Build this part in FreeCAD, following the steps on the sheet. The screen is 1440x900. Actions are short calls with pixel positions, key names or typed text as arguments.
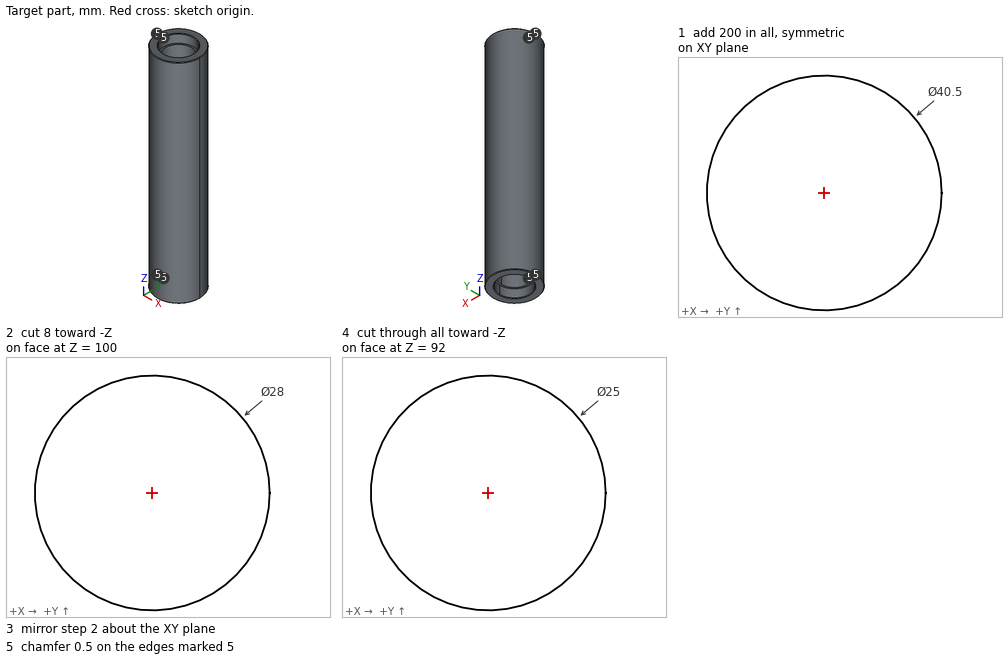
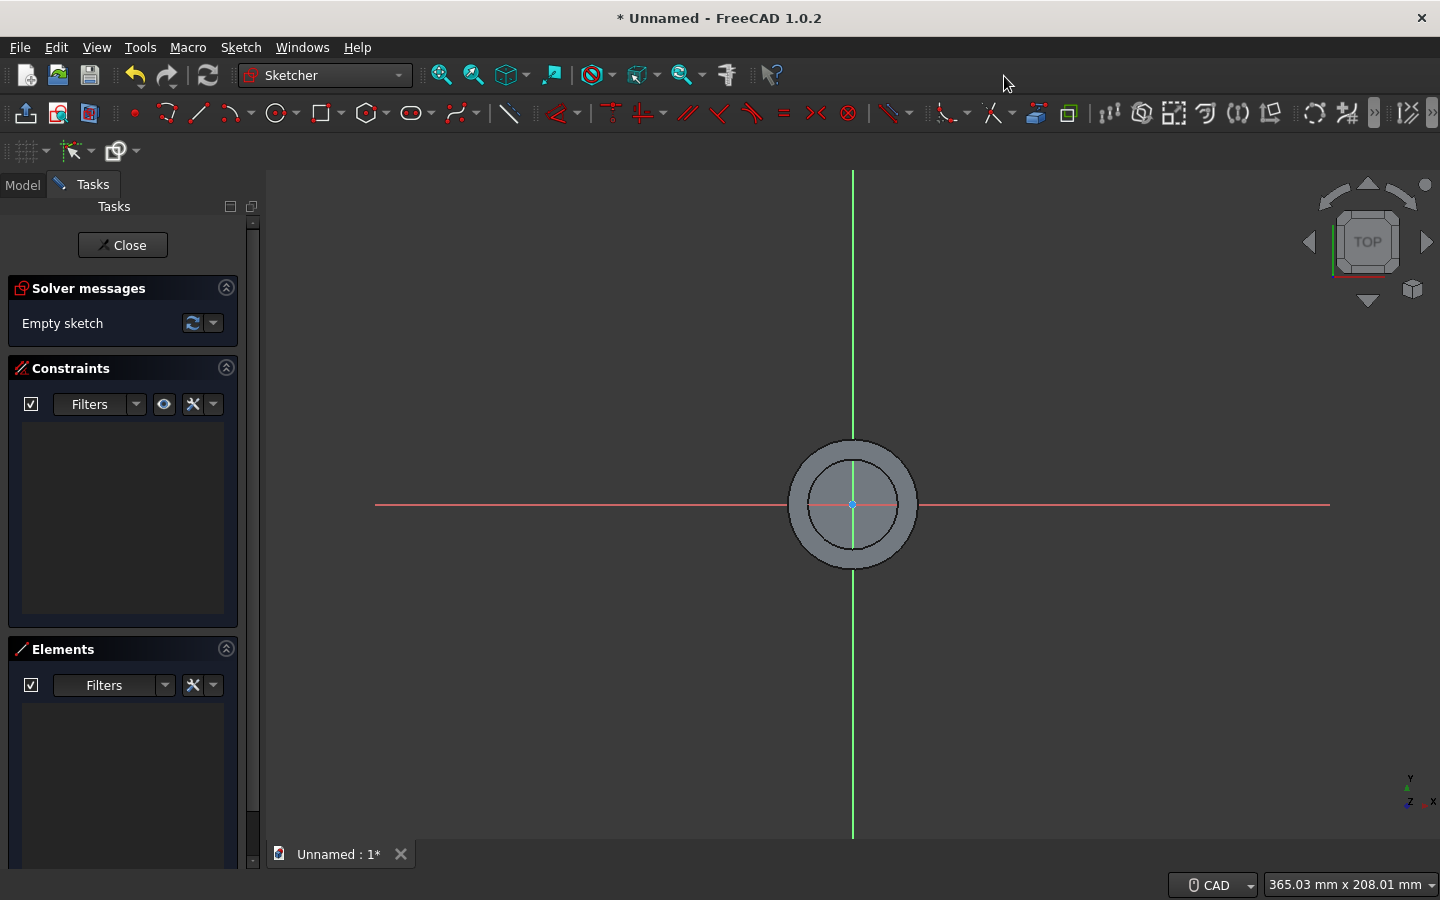
scroll(870, 504, up, 8)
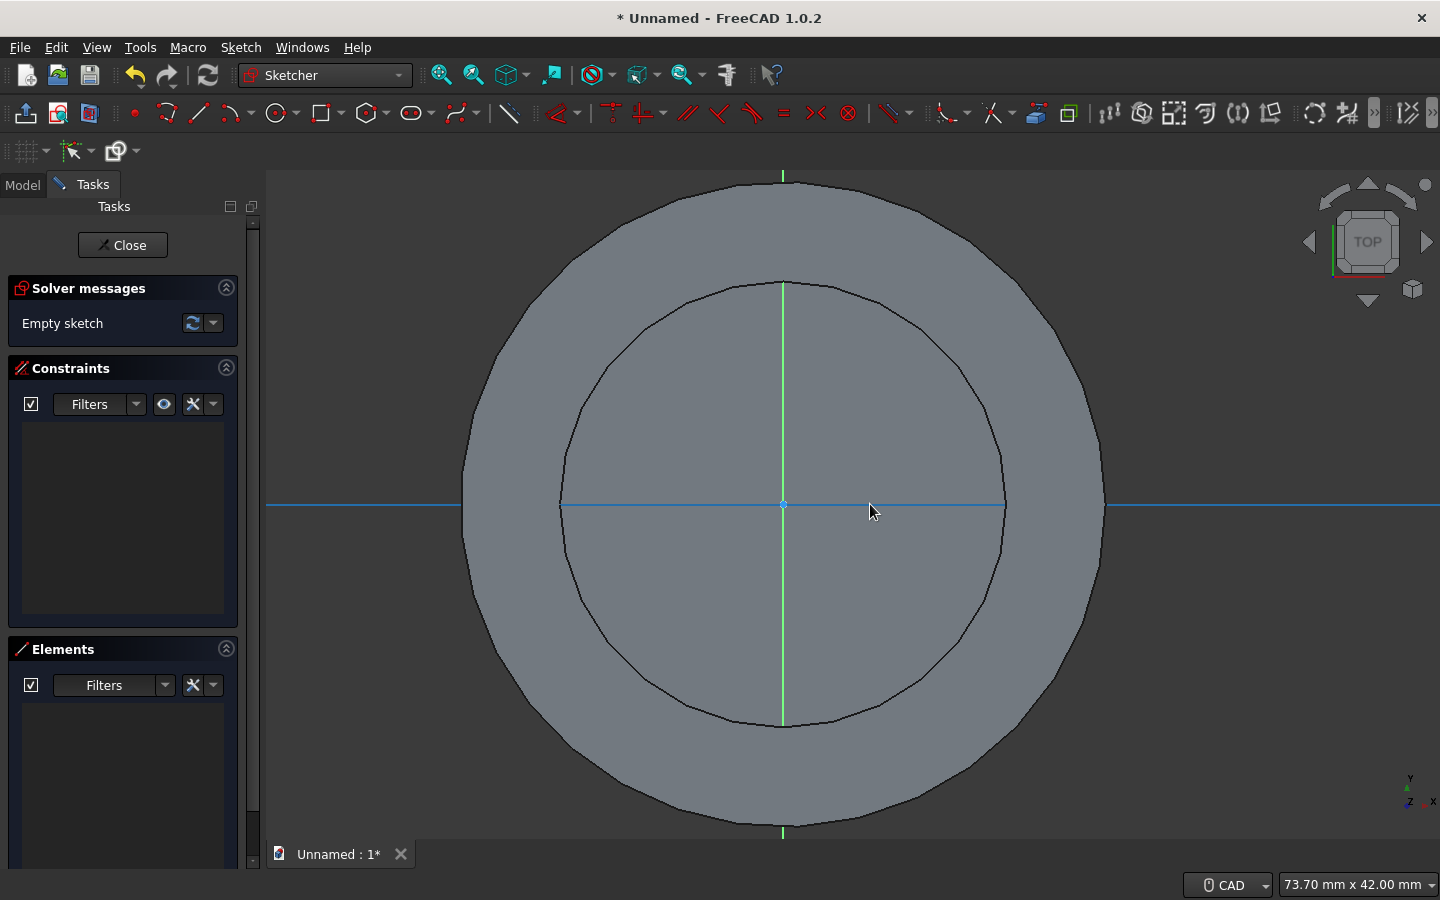
click(276, 114)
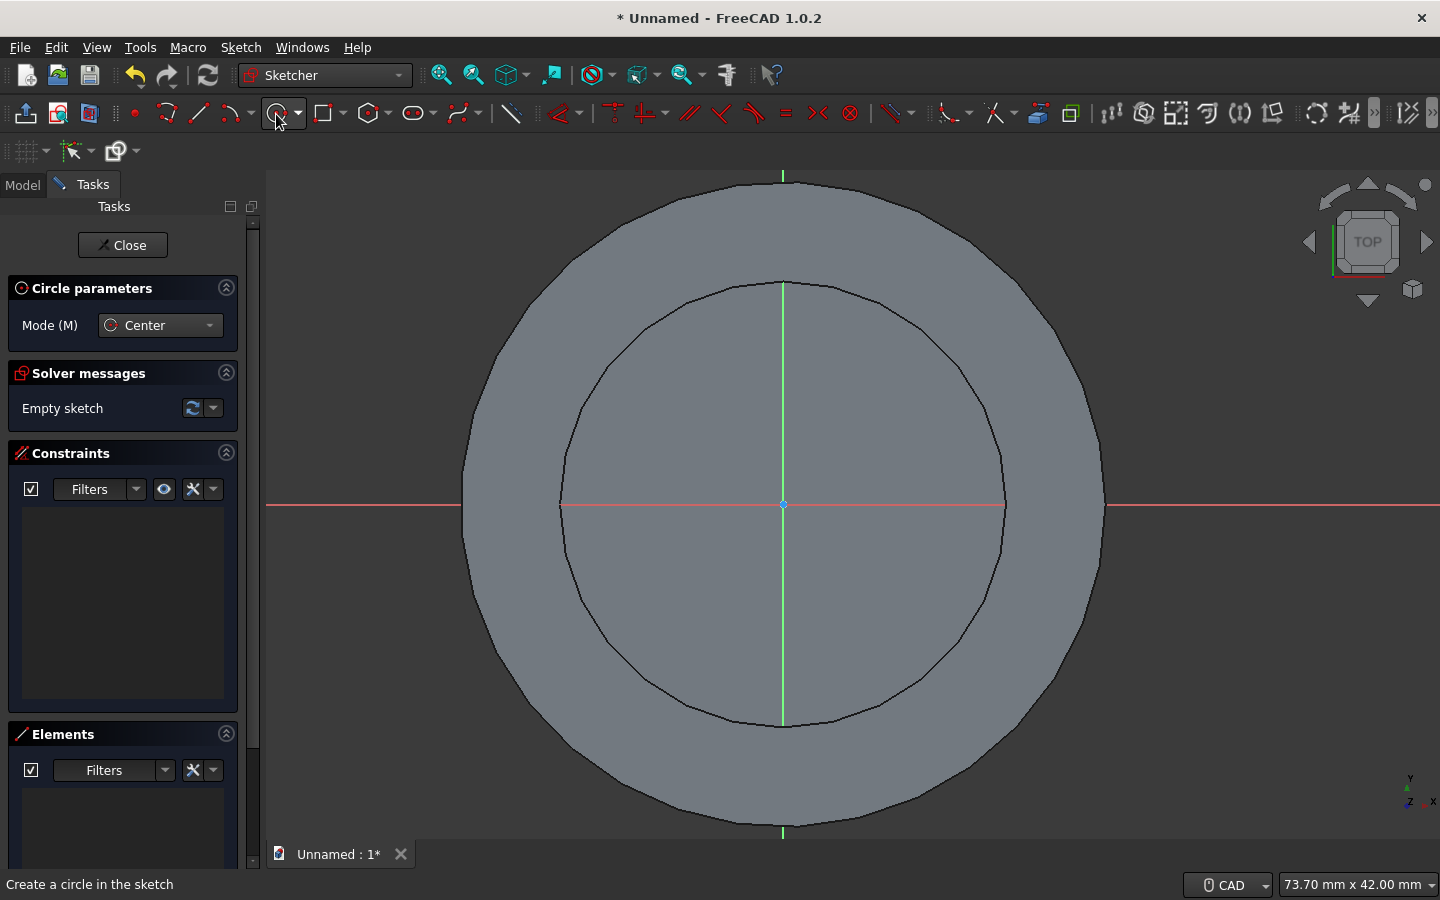
click(783, 504)
move(924, 364)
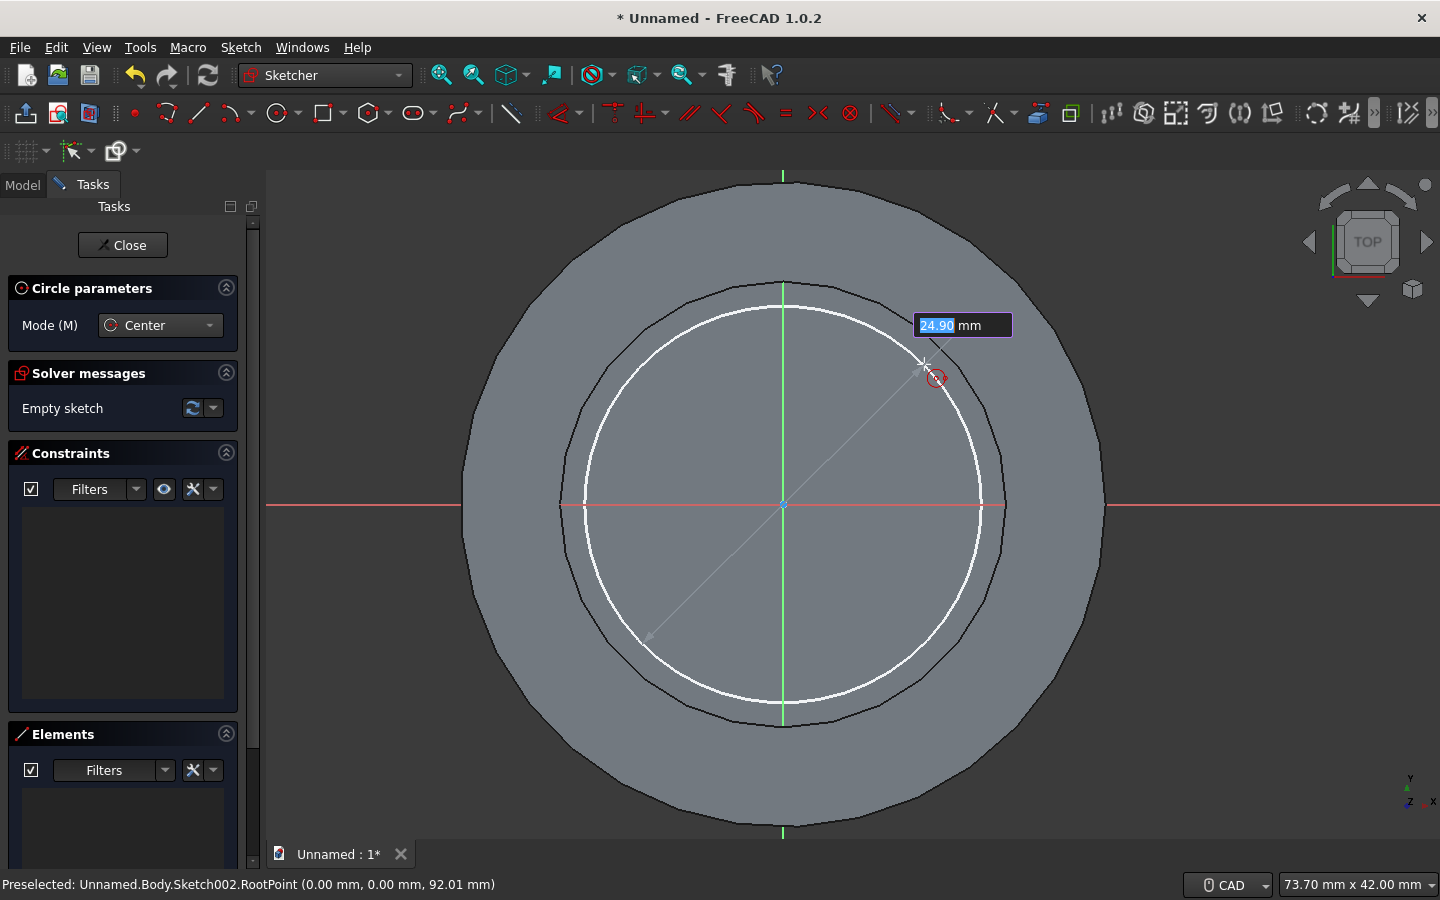
text(25)
key(Return)
key(Escape)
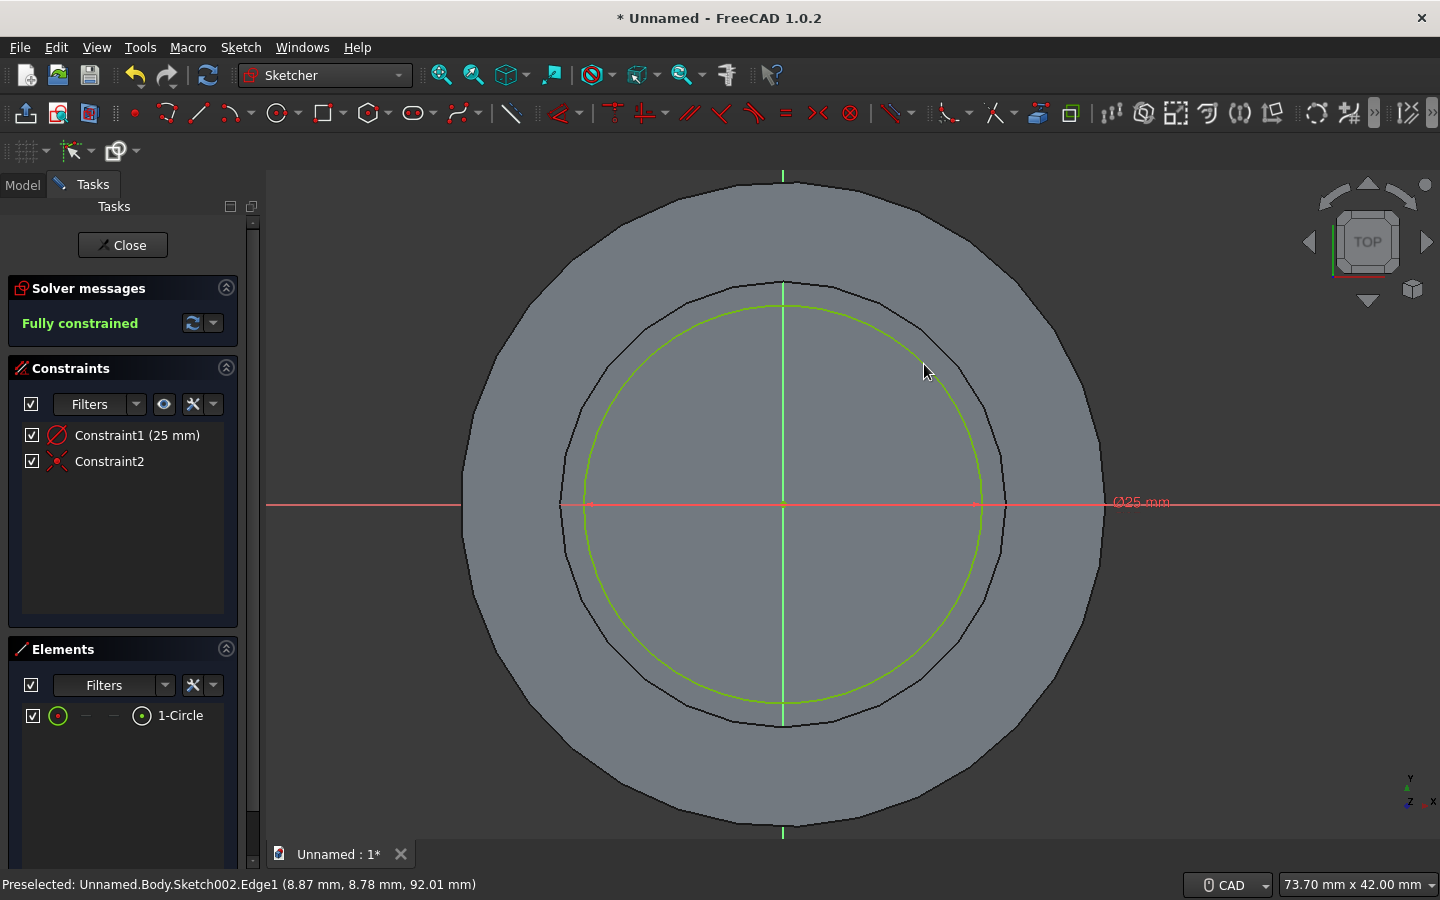
click(123, 245)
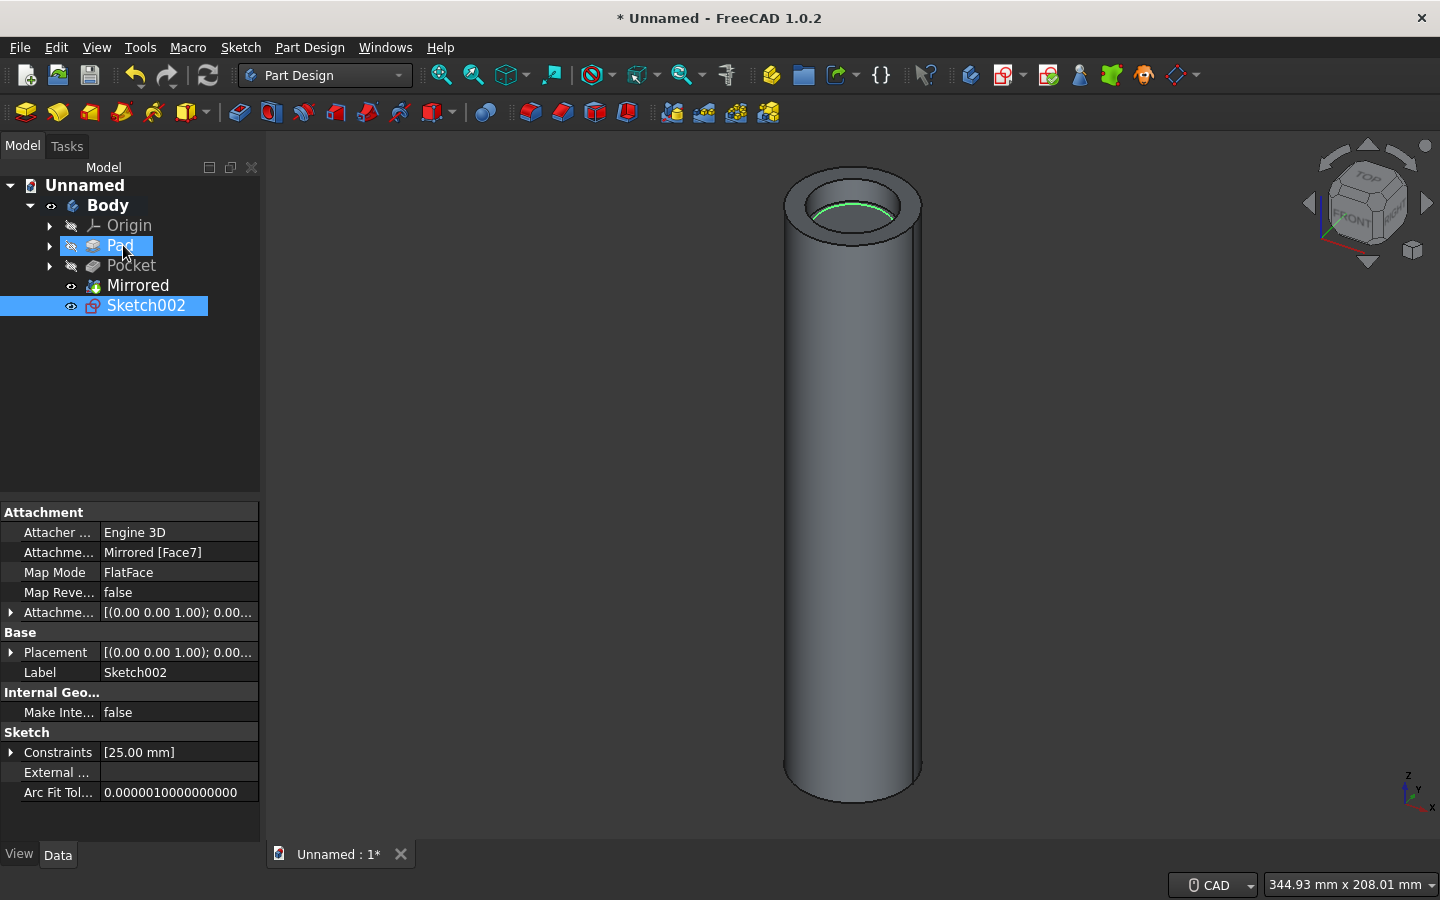
click(240, 112)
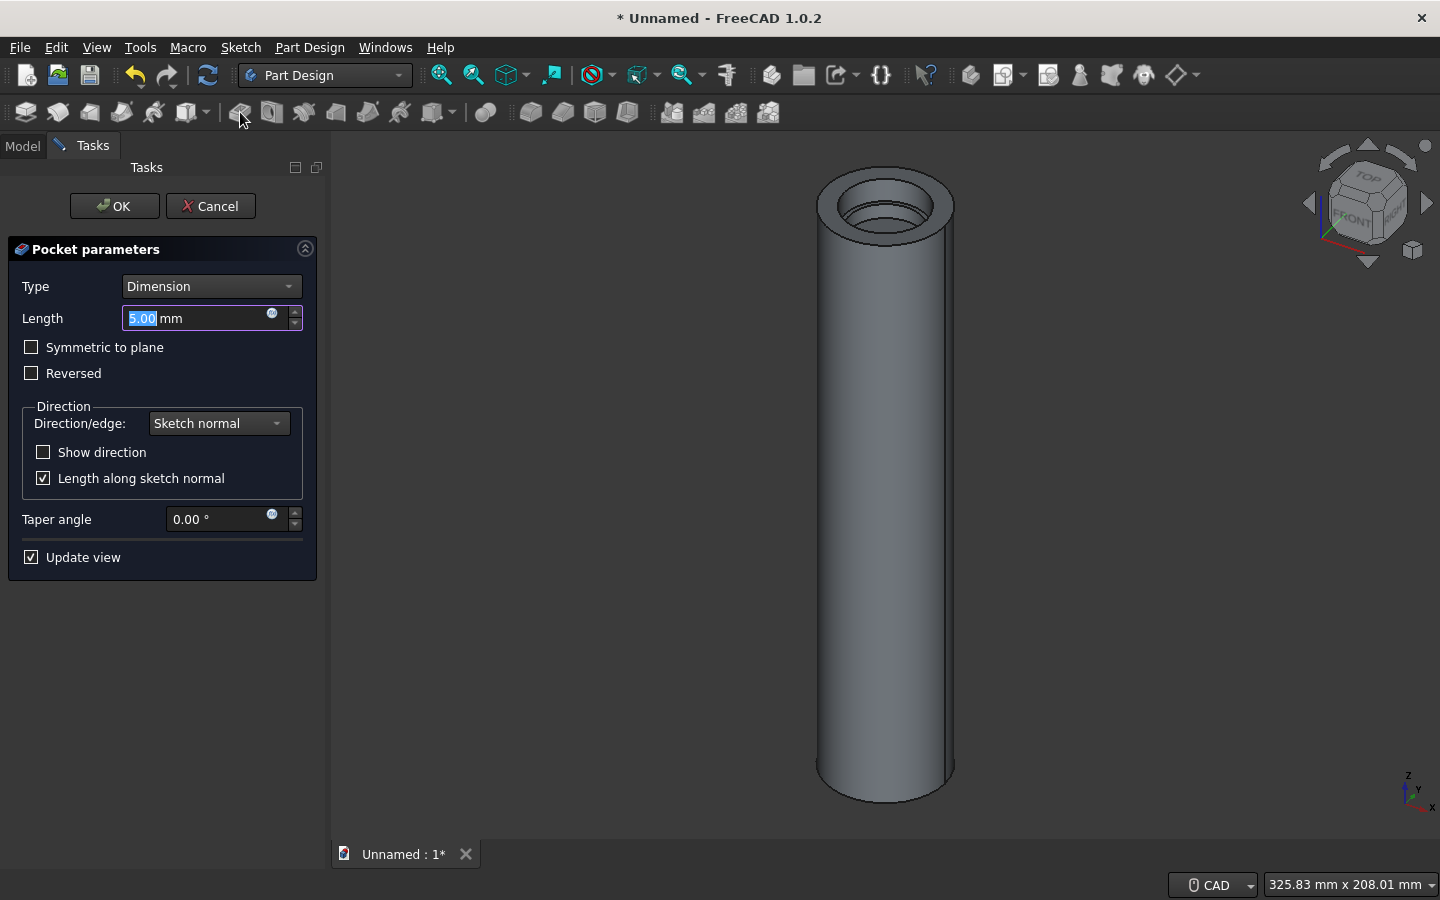
click(212, 286)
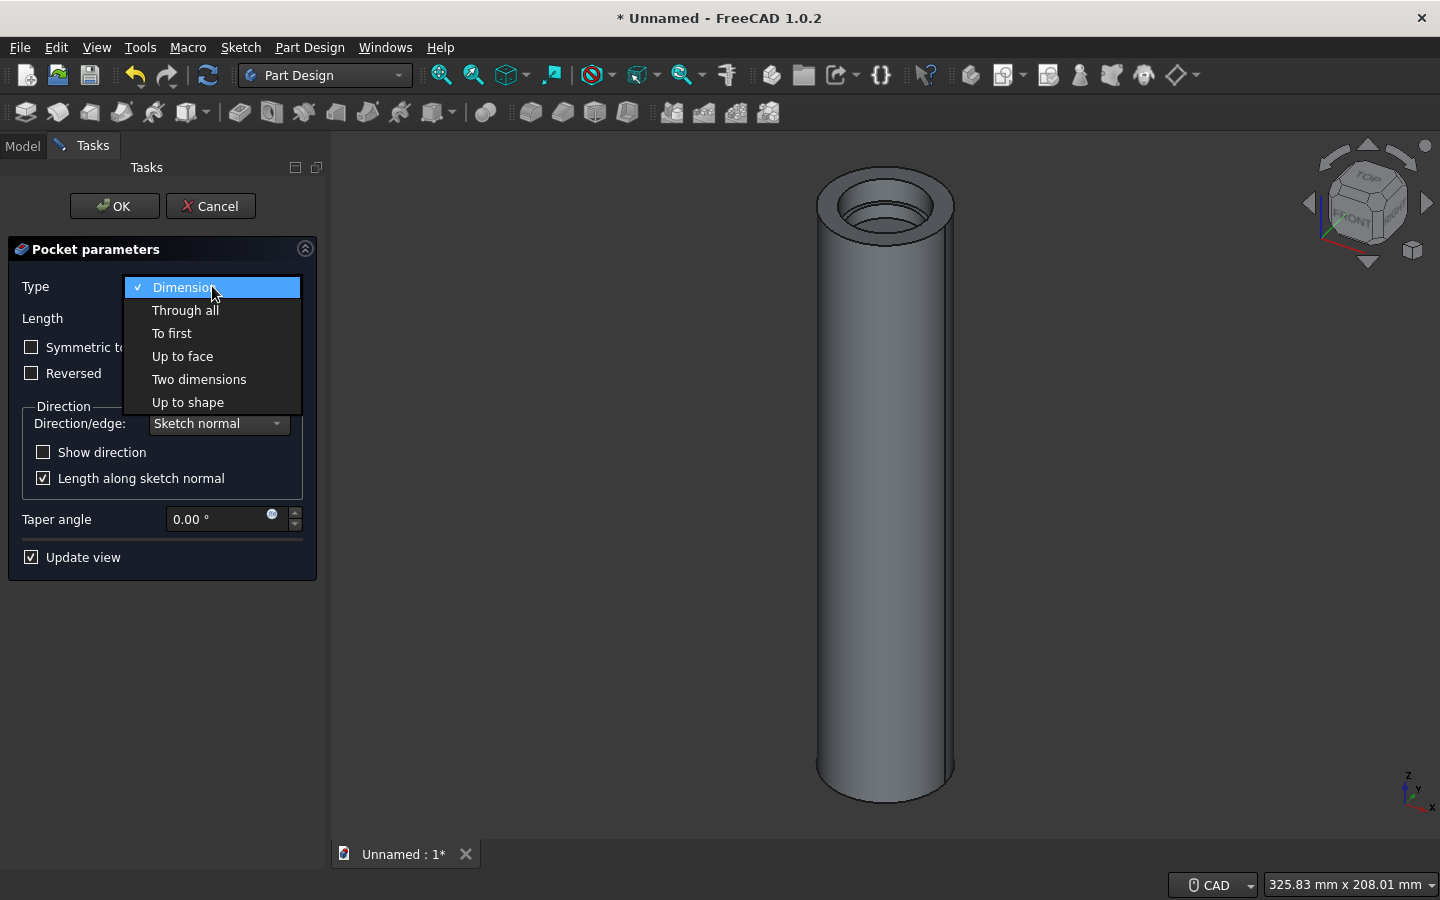
click(212, 310)